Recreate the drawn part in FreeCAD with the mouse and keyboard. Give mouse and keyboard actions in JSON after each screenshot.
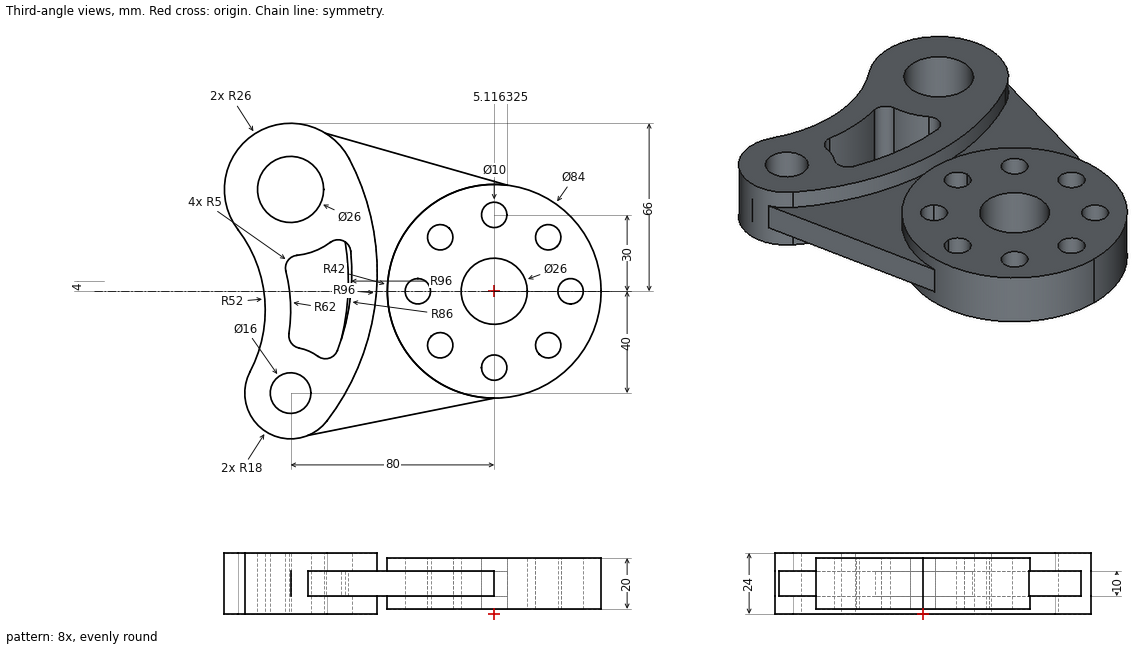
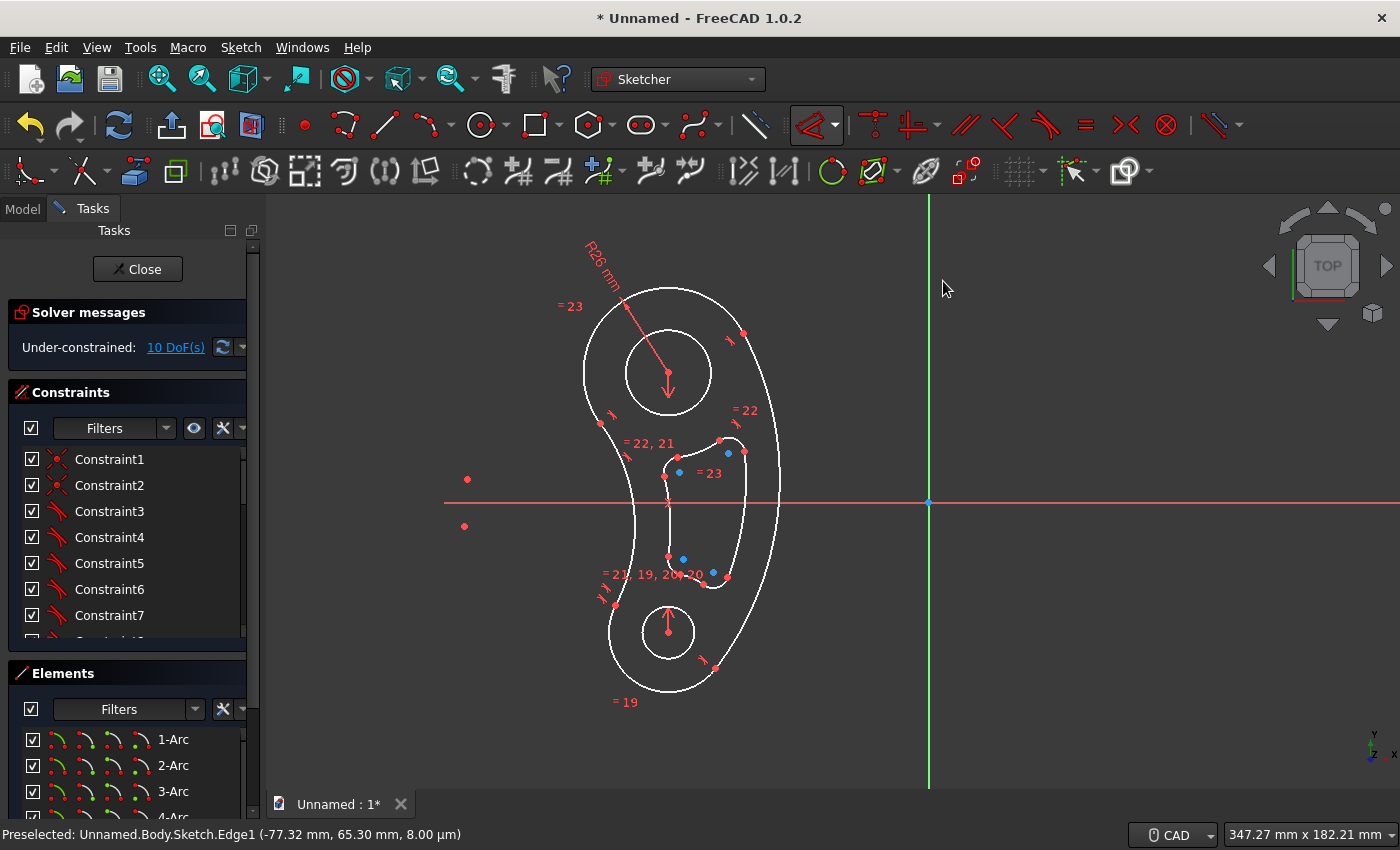
{"action": "left_click", "coordinate": [633, 551]}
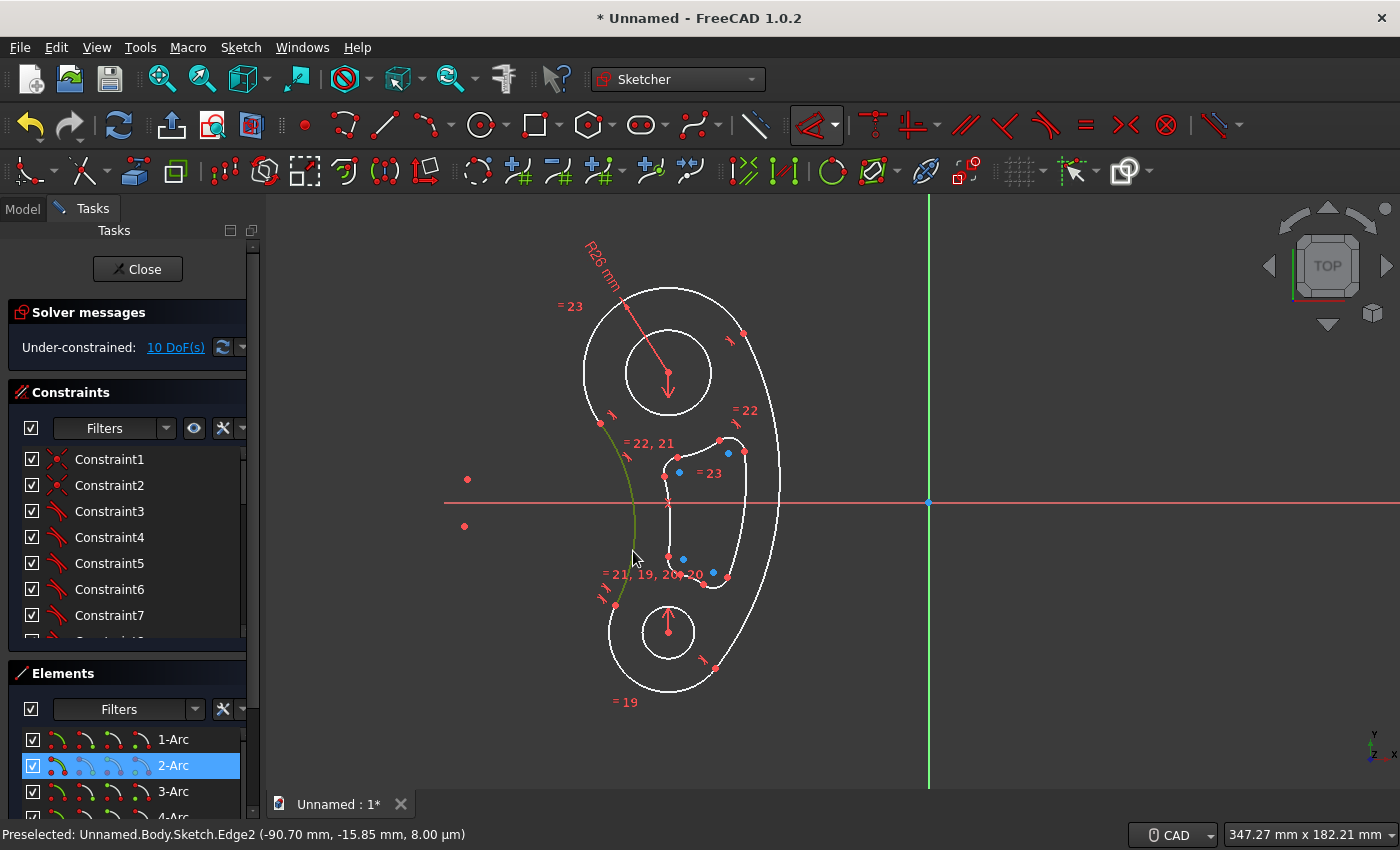
{"action": "left_click", "coordinate": [838, 126]}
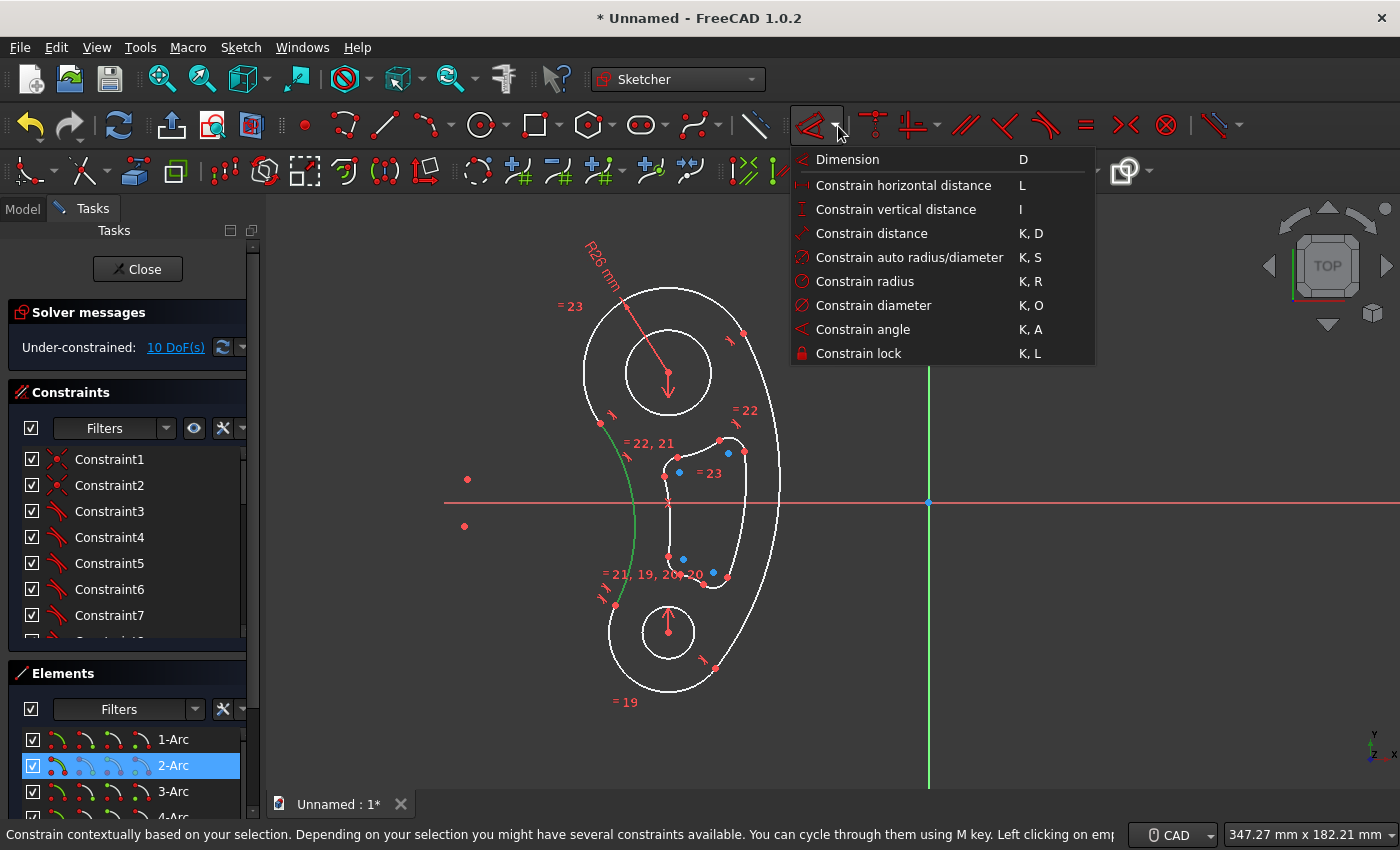
{"action": "left_click", "coordinate": [943, 281]}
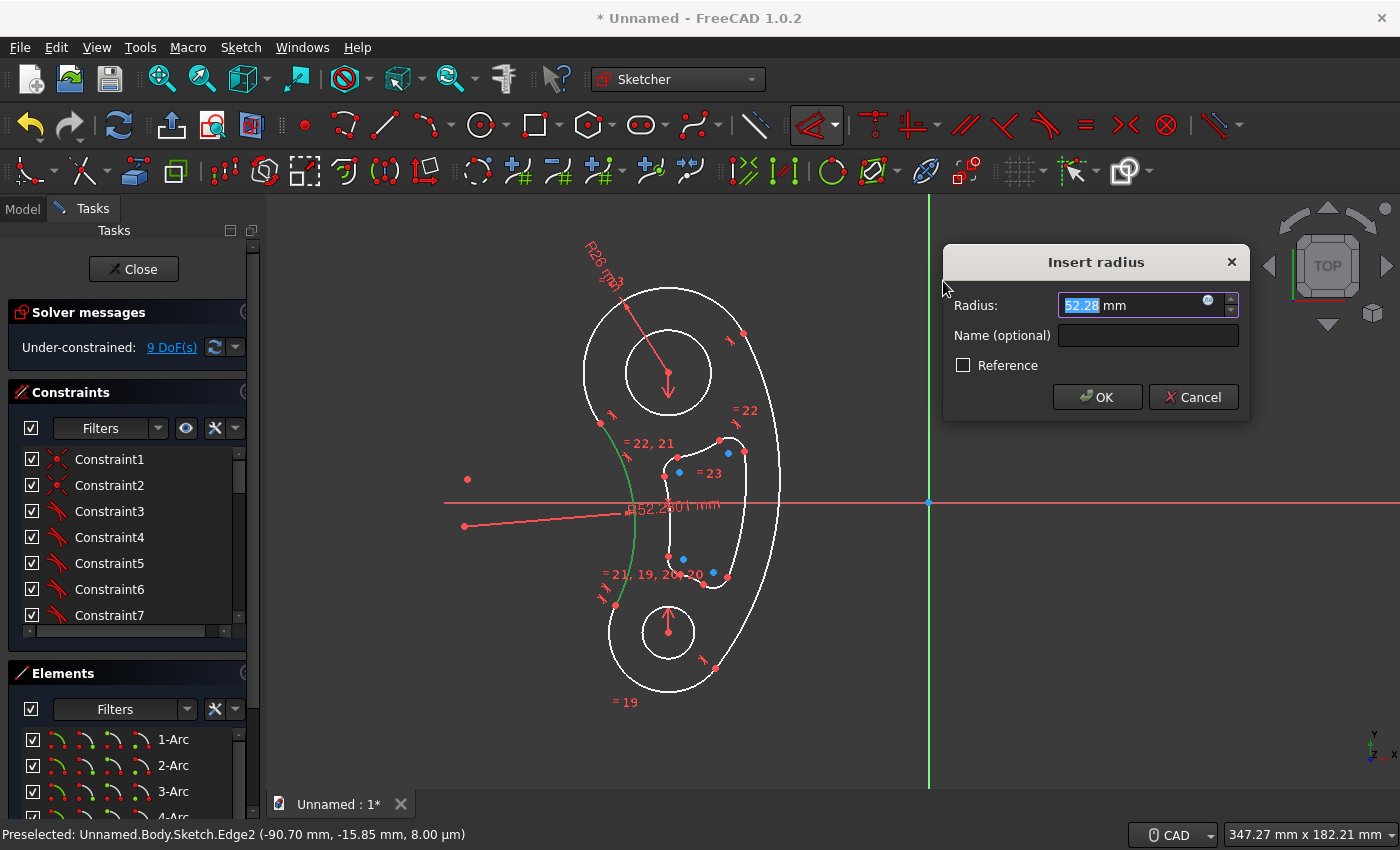
{"action": "type", "text": "52"}
{"action": "key", "text": "Return"}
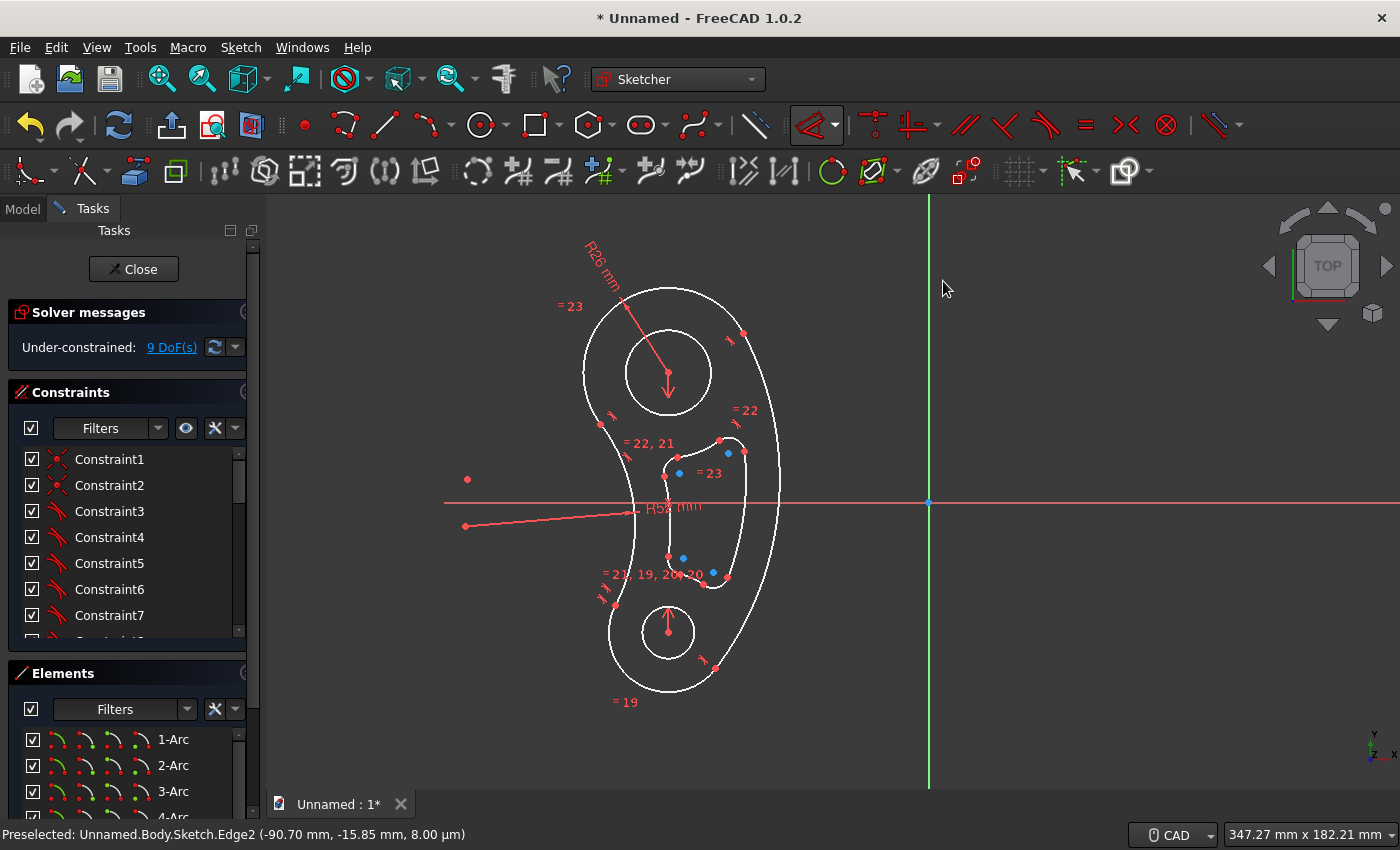
{"action": "left_click", "coordinate": [614, 656]}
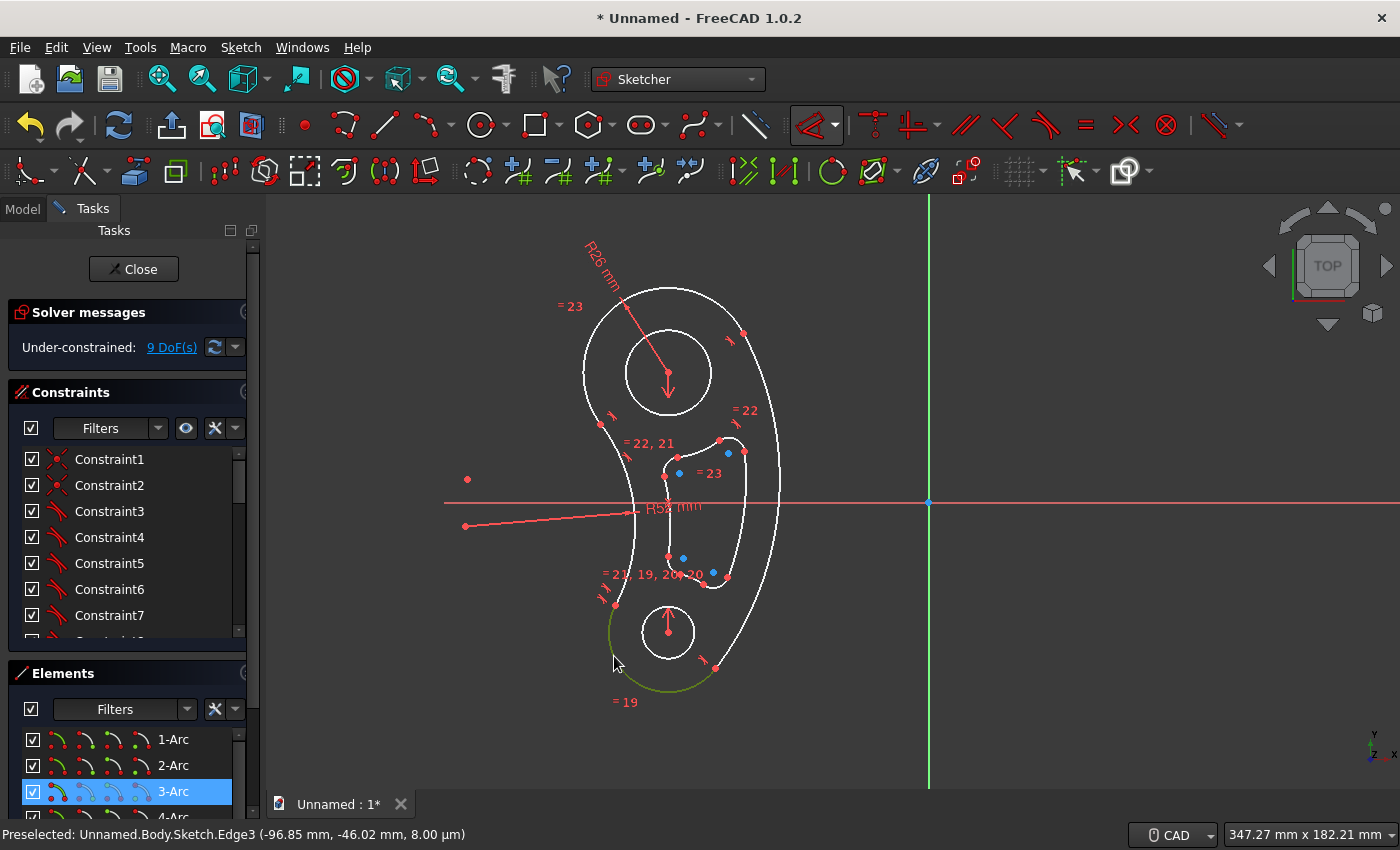
{"action": "key", "text": "k r"}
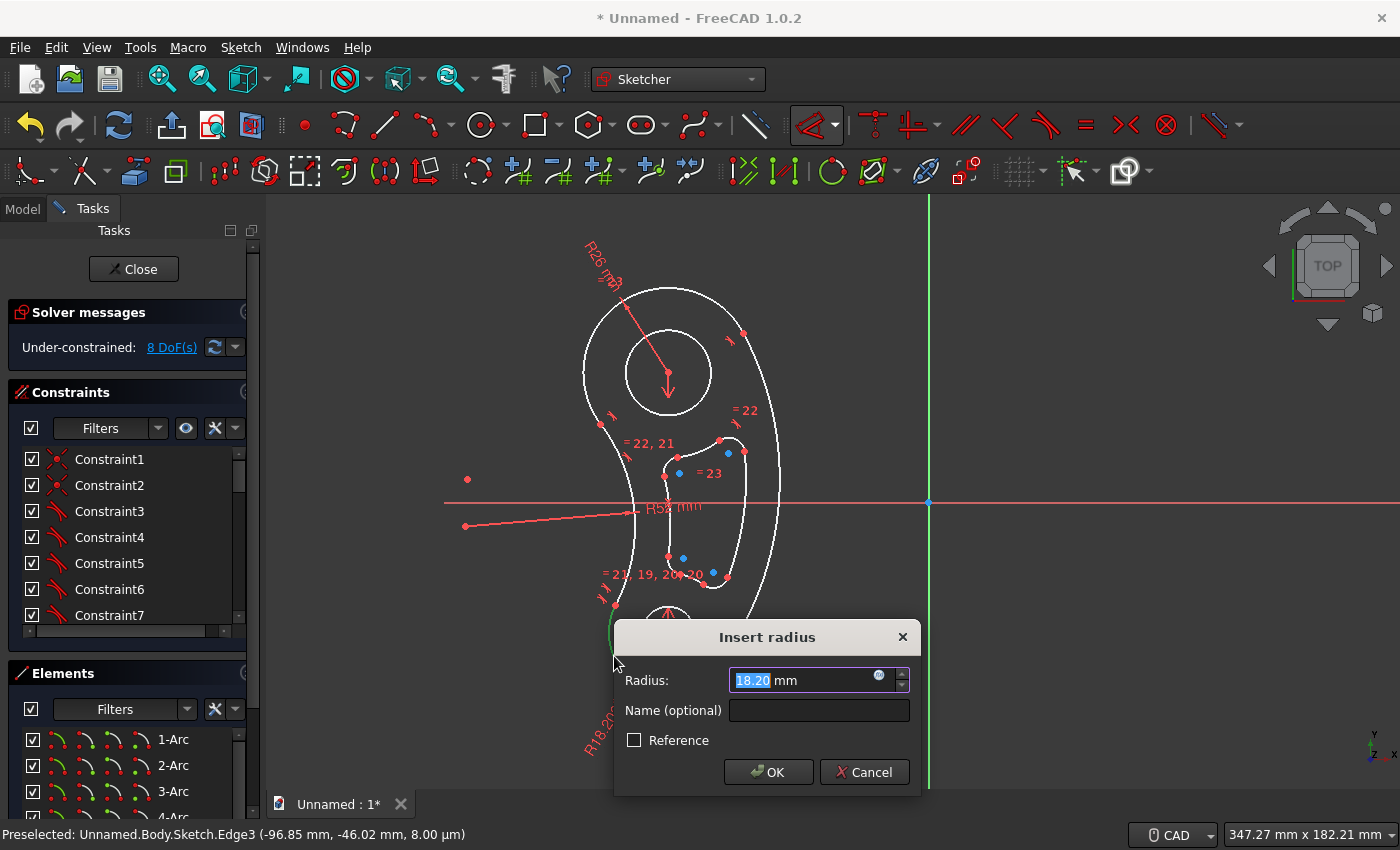
{"action": "type", "text": "18"}
{"action": "key", "text": "Return"}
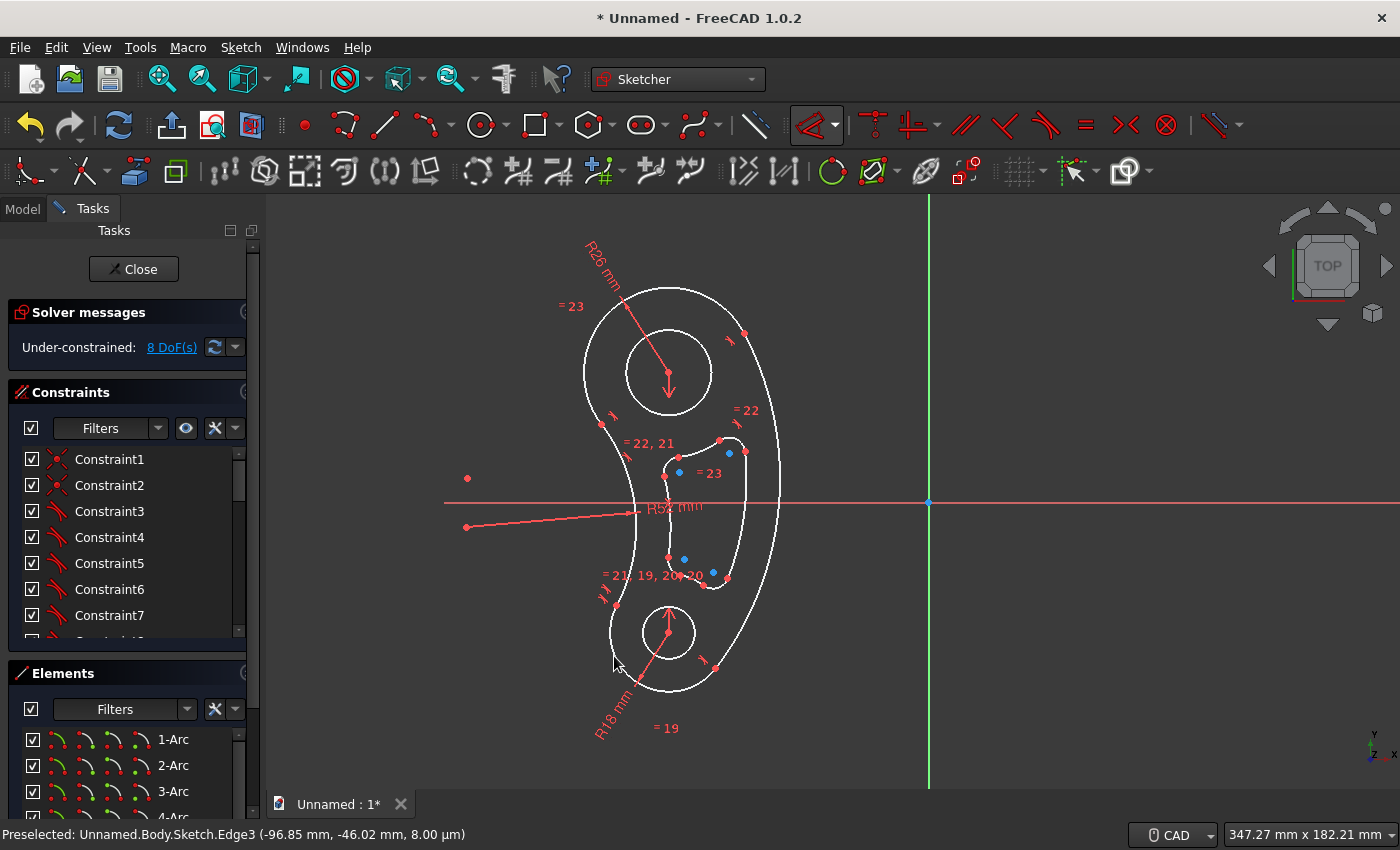
{"action": "left_click", "coordinate": [765, 575]}